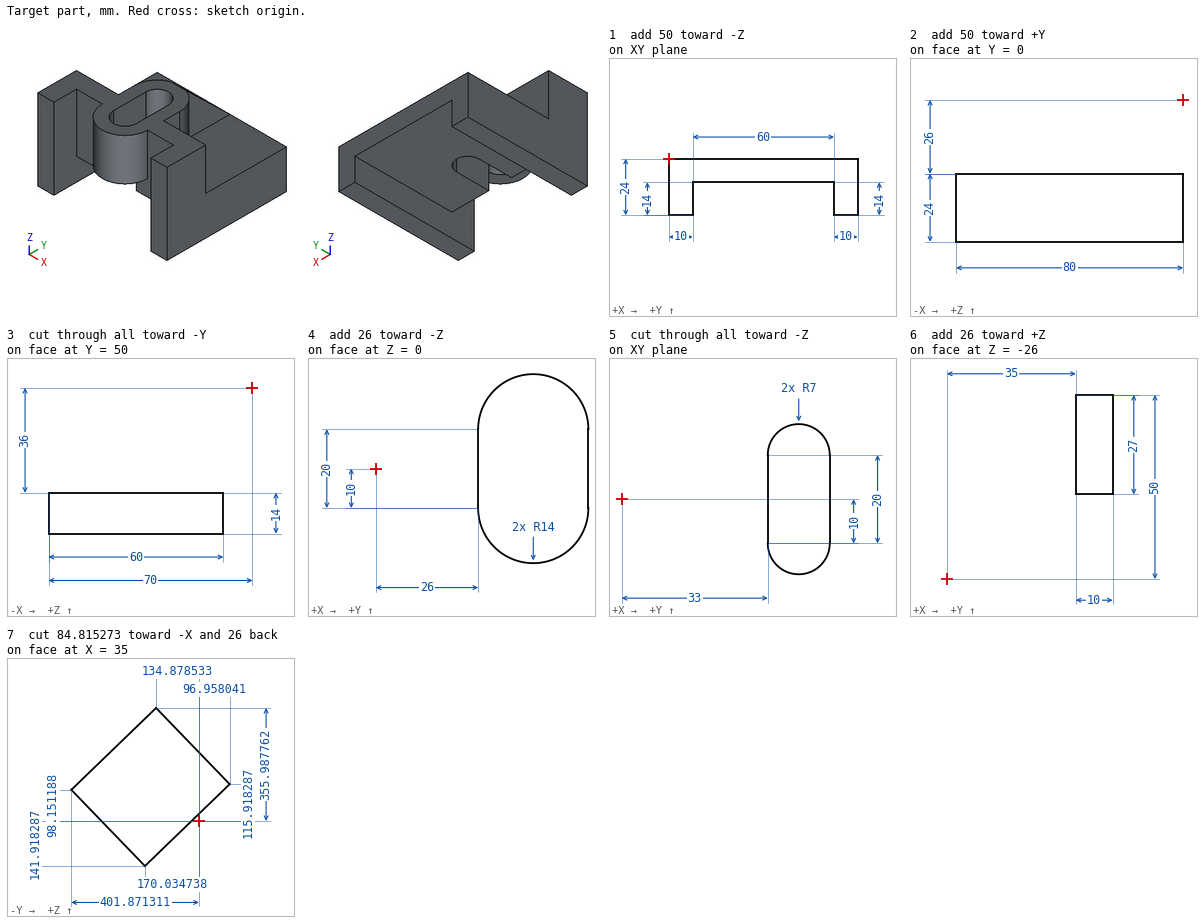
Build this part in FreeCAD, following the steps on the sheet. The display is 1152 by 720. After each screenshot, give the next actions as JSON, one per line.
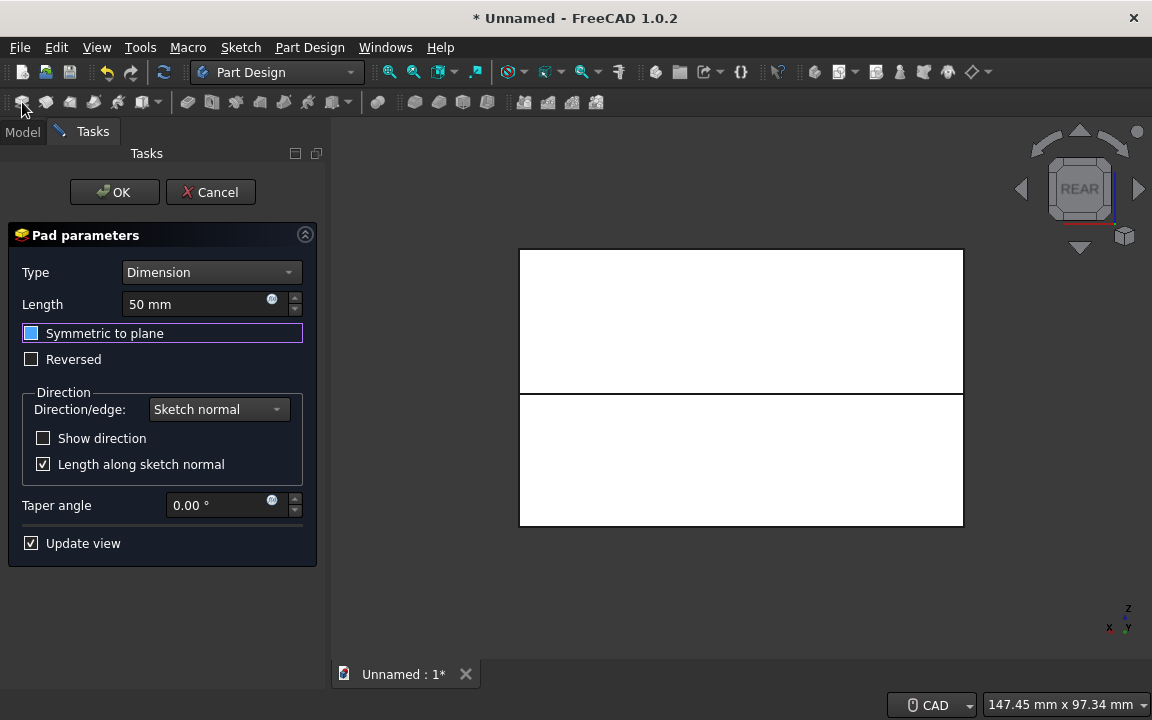
{"action": "left_click", "coordinate": [115, 192]}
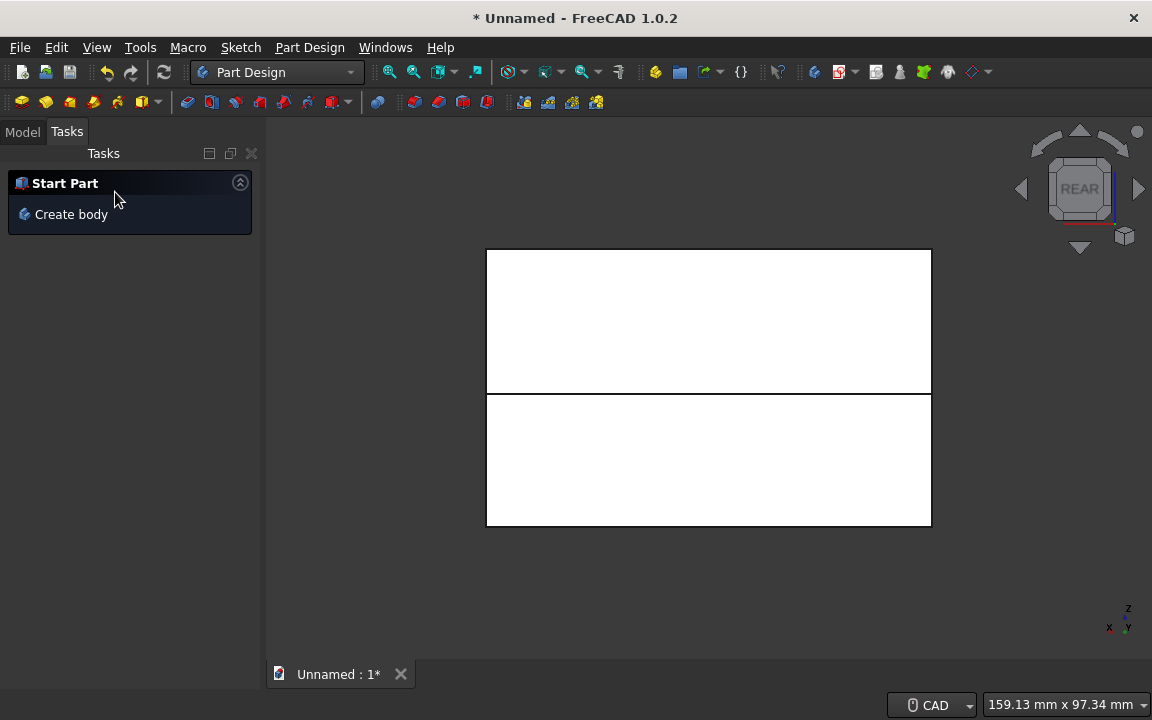
{"action": "left_click", "coordinate": [582, 459]}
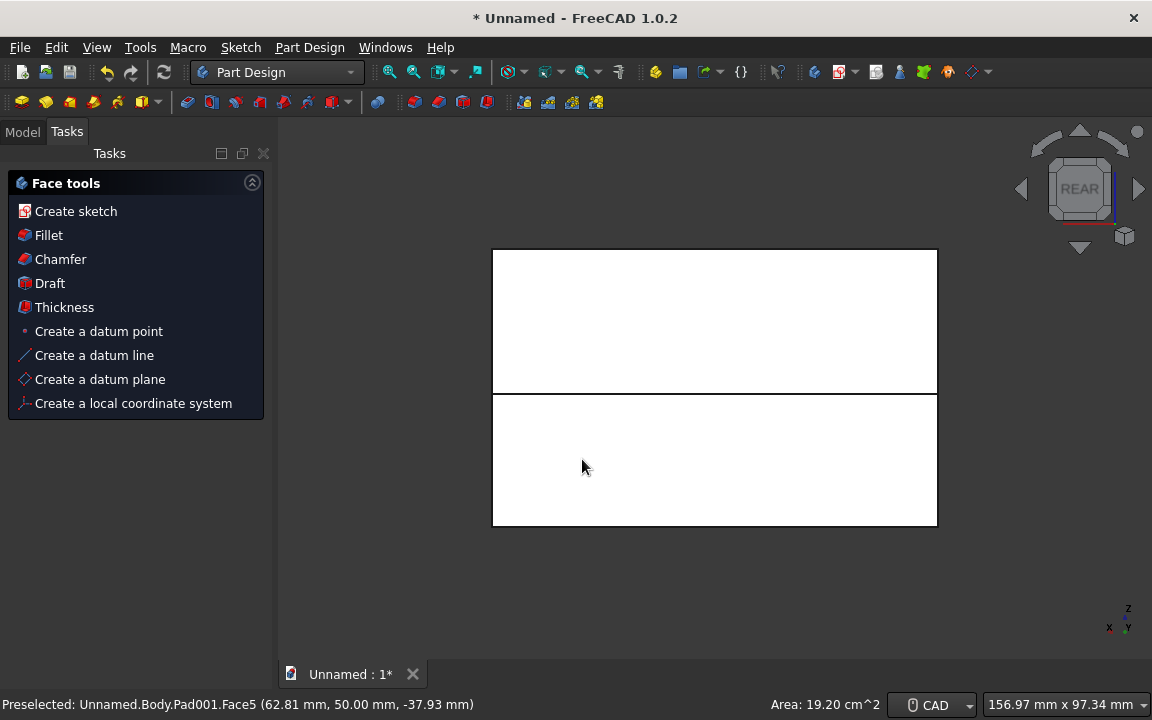
{"action": "left_click", "coordinate": [840, 72]}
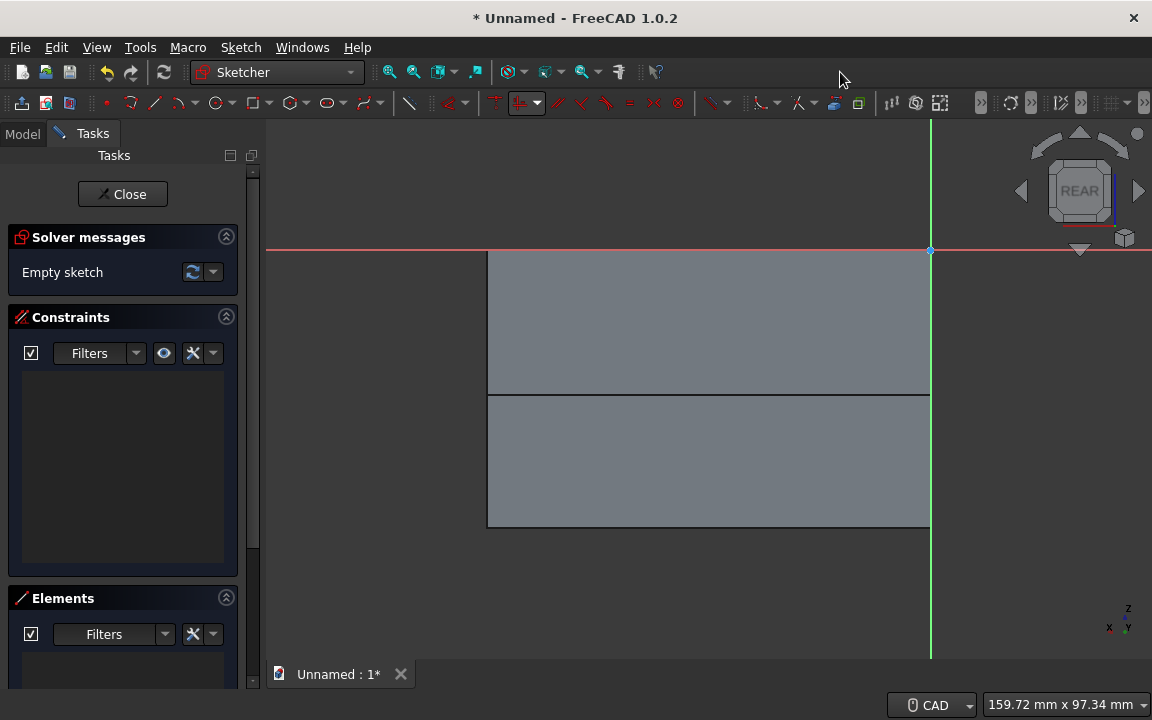
{"action": "key", "text": "g r"}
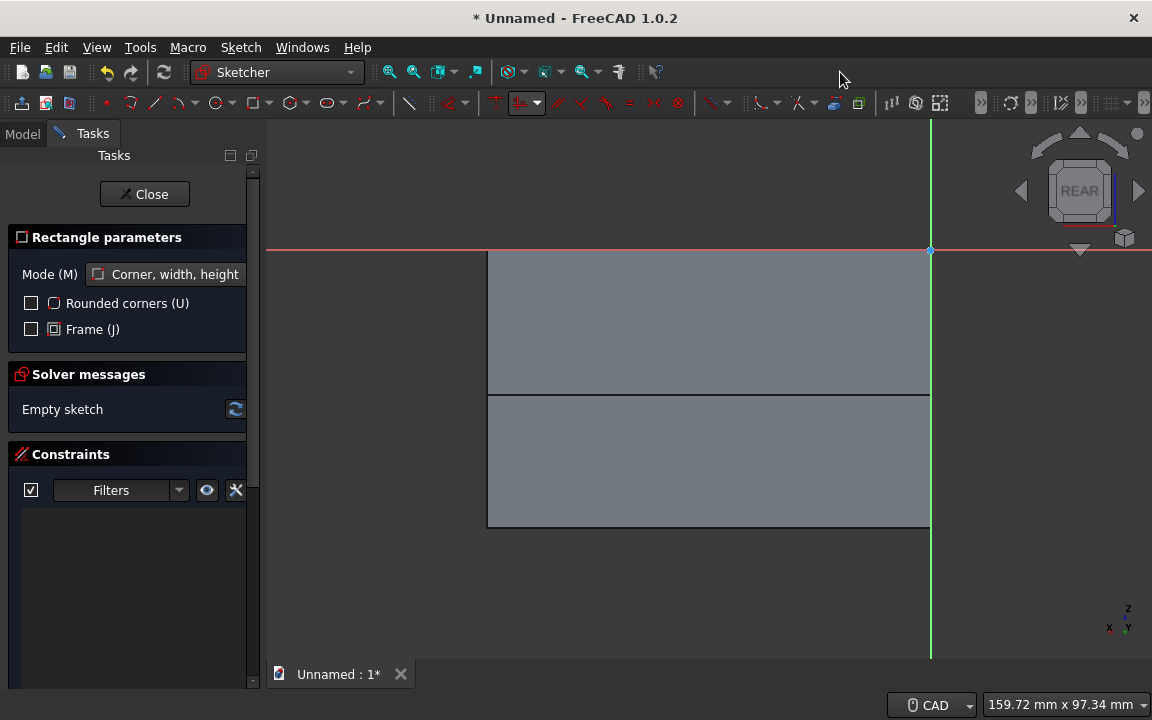
{"action": "left_click", "coordinate": [543, 450]}
{"action": "mouse_move", "coordinate": [875, 528]}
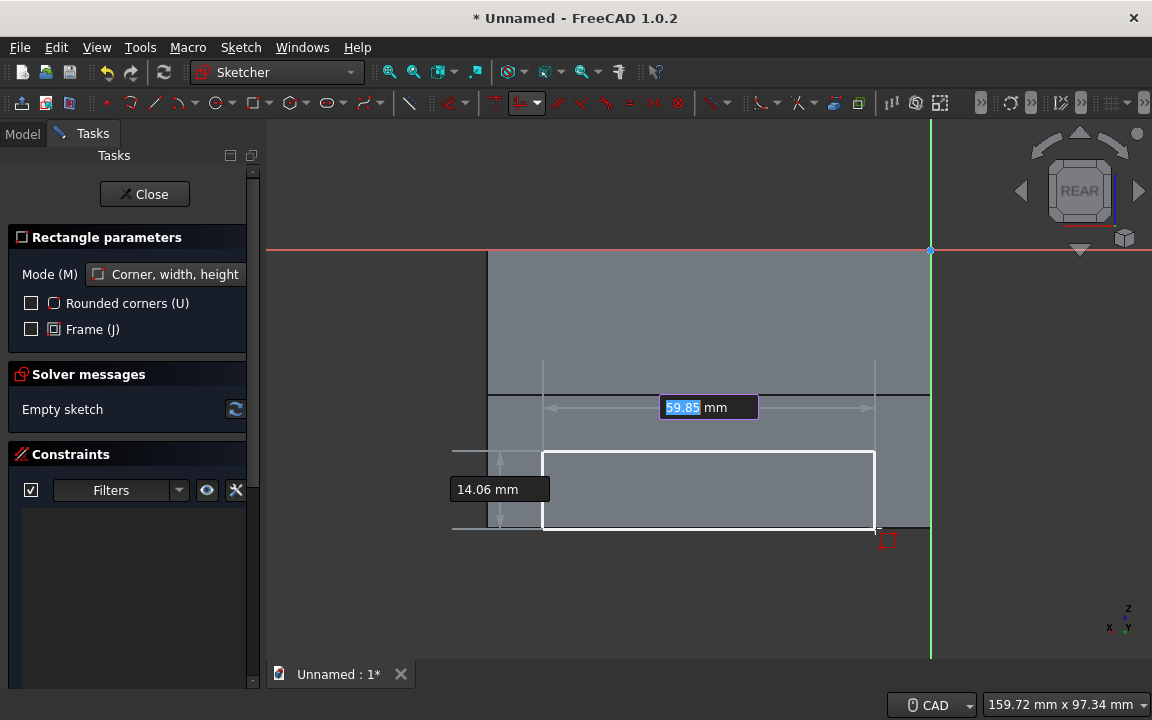
{"action": "type", "text": "60"}
{"action": "key", "text": "Tab"}
{"action": "type", "text": "14"}
{"action": "key", "text": "Return"}
{"action": "key", "text": "Escape"}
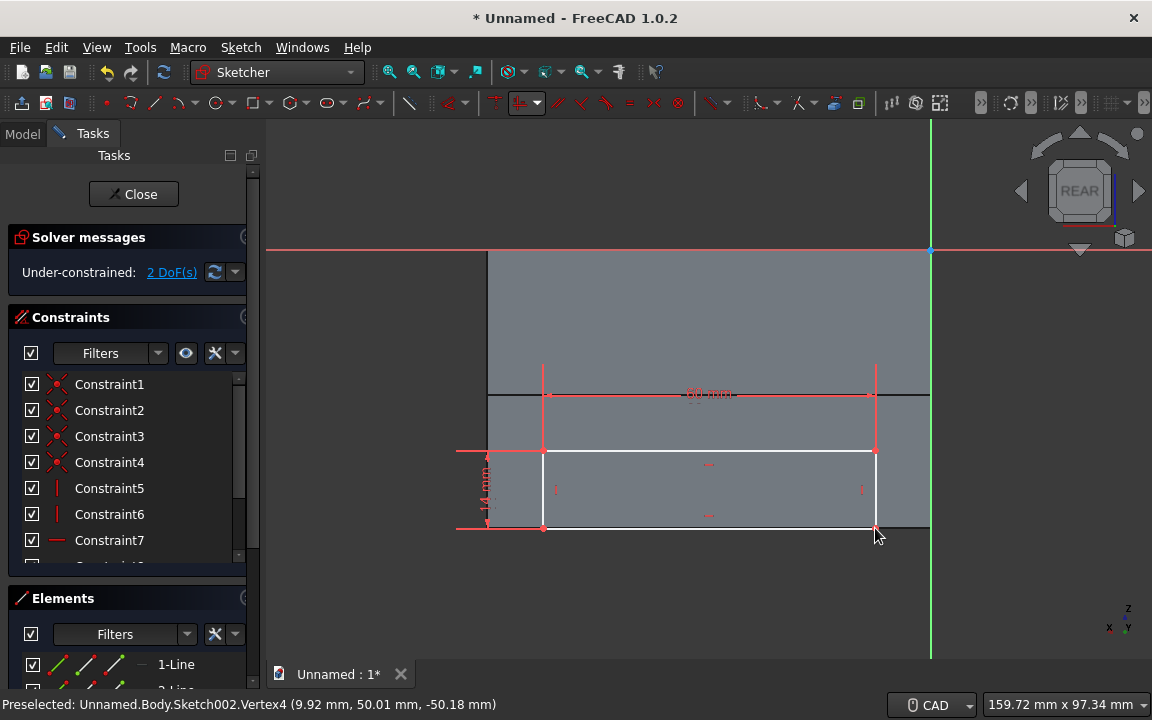
{"action": "key", "text": "d"}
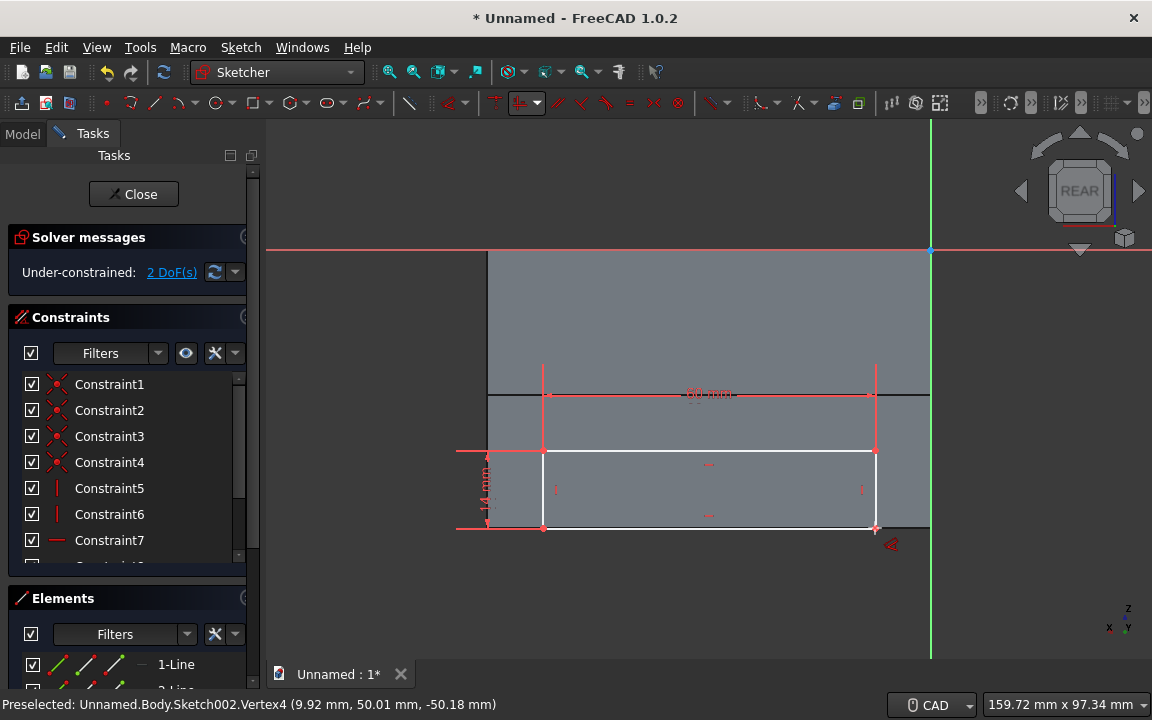
{"action": "left_click", "coordinate": [543, 451]}
{"action": "left_click", "coordinate": [737, 216]}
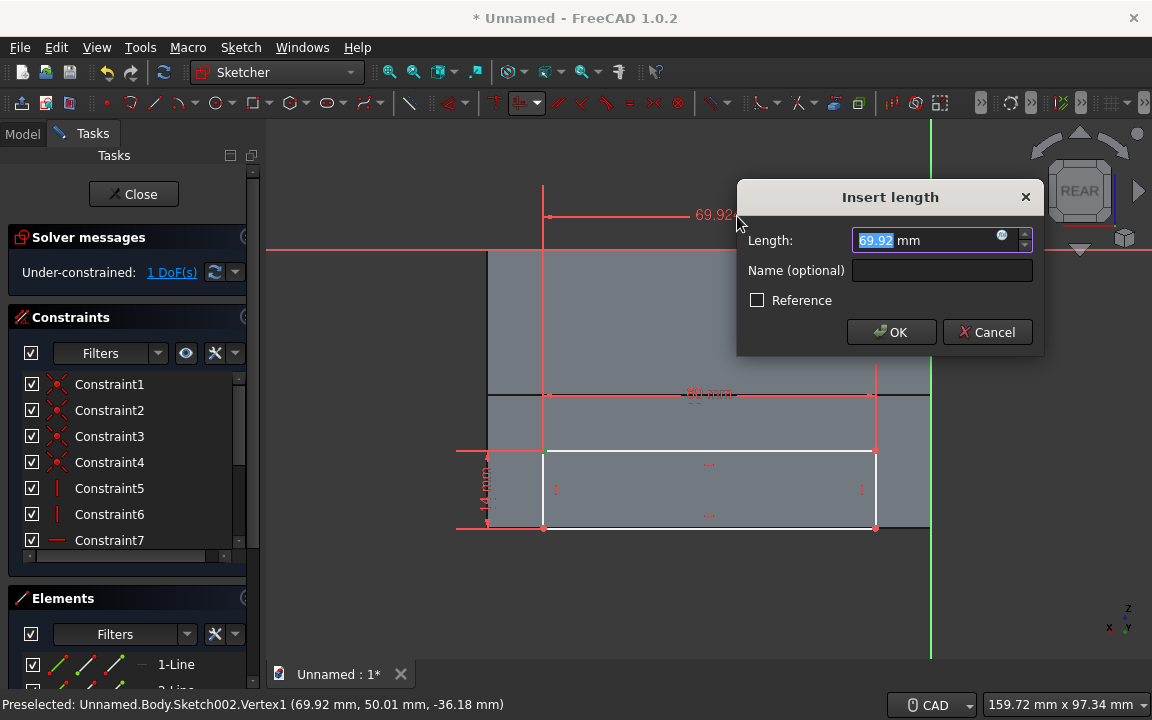
{"action": "type", "text": "70"}
{"action": "key", "text": "Return"}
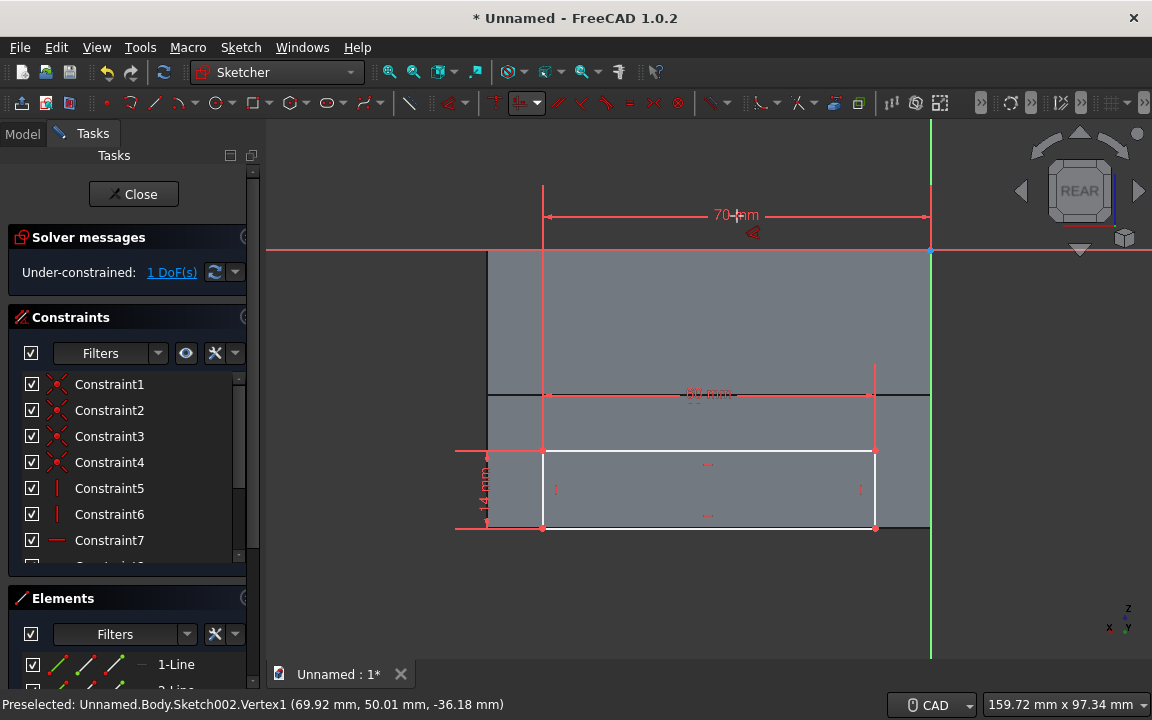
{"action": "left_click", "coordinate": [543, 451]}
{"action": "left_click", "coordinate": [965, 351]}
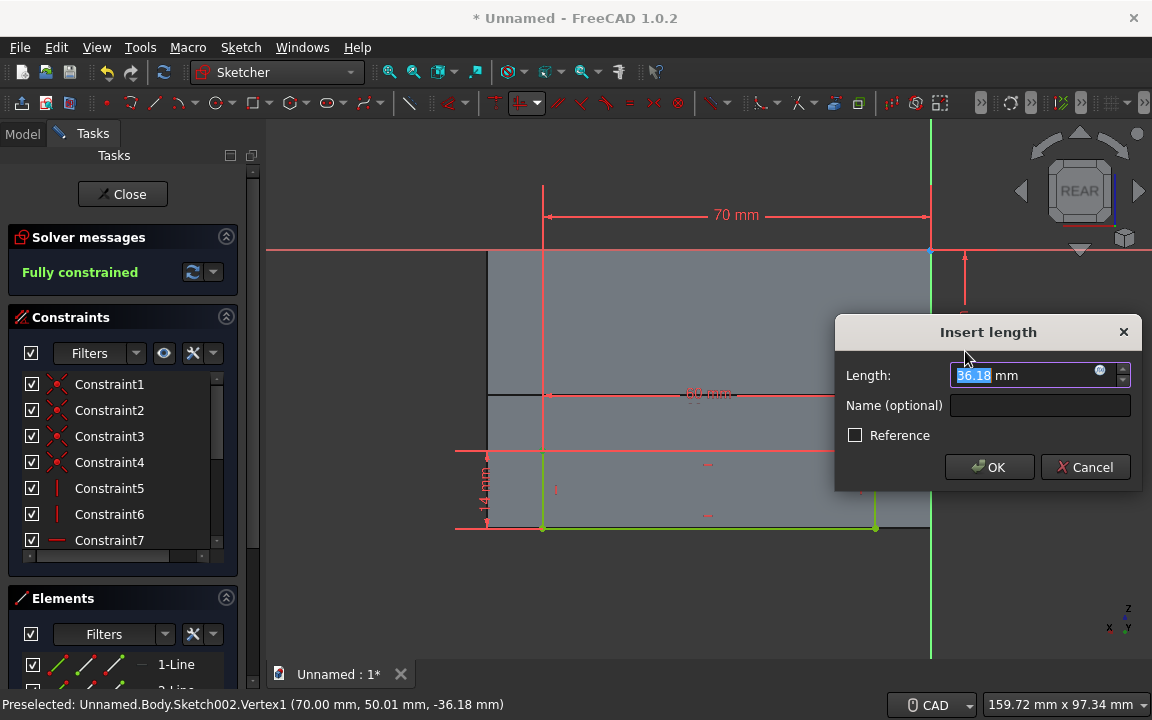
{"action": "type", "text": "36"}
{"action": "key", "text": "Return"}
{"action": "key", "text": "Escape"}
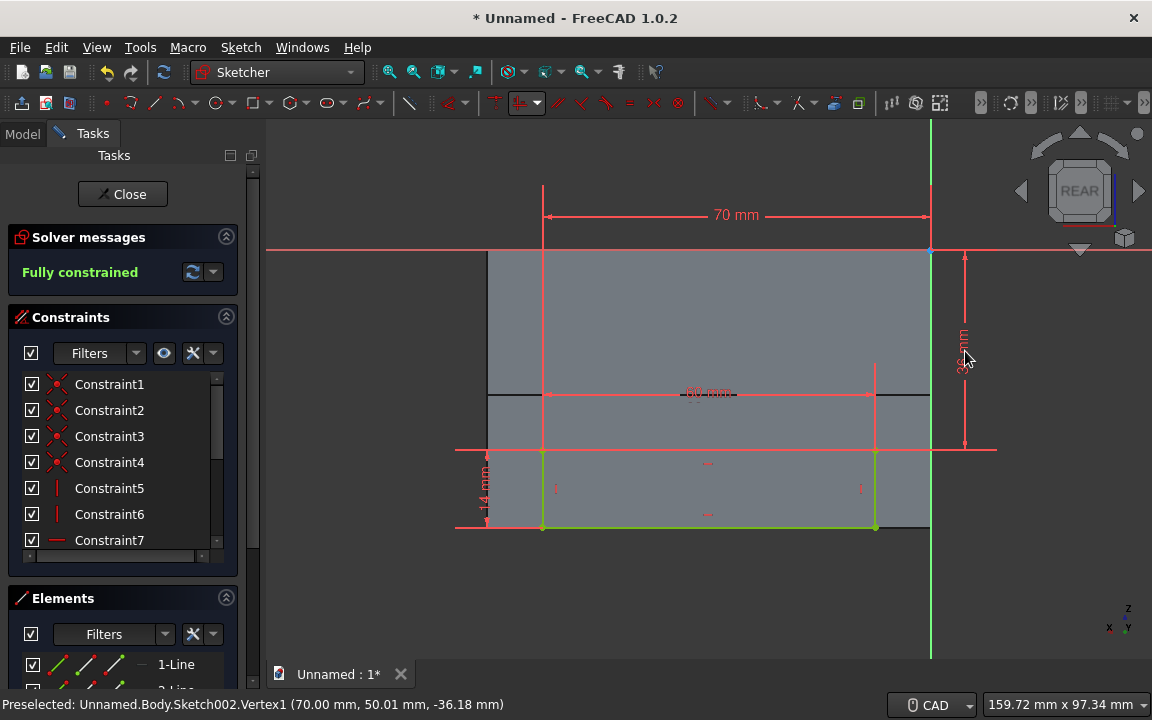
{"action": "left_click", "coordinate": [123, 194]}